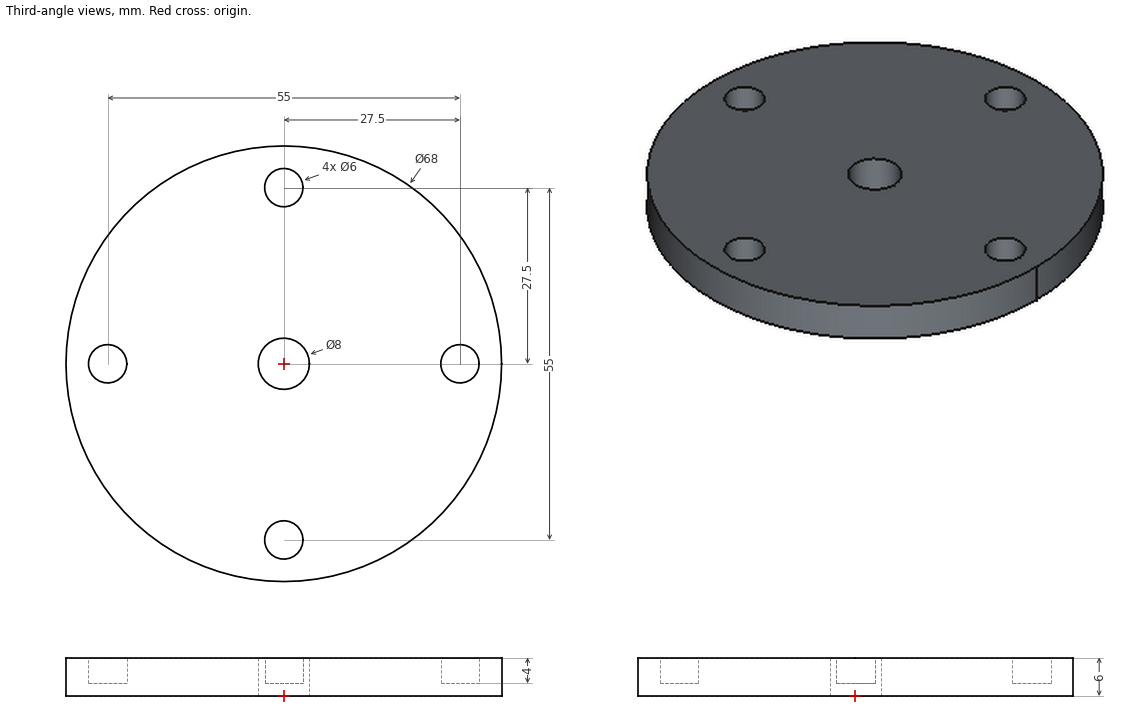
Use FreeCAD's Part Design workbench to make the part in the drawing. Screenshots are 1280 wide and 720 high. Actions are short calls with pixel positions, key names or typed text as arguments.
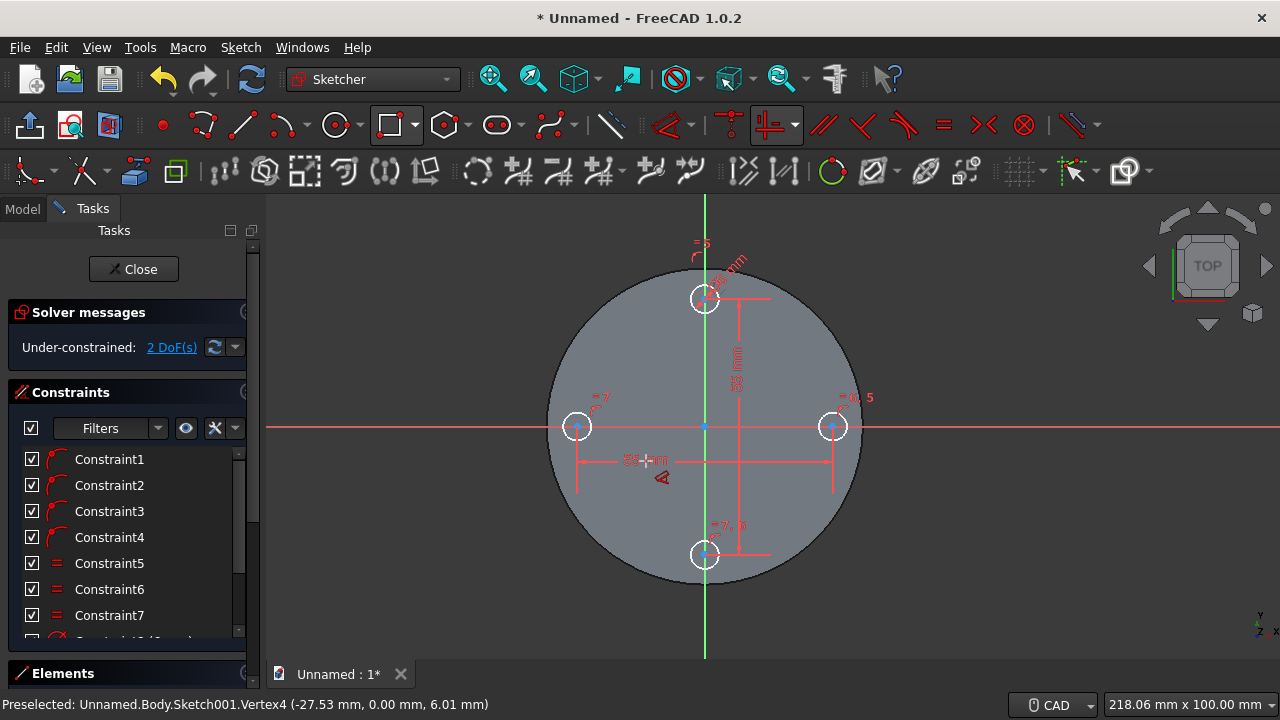
click(705, 299)
click(739, 334)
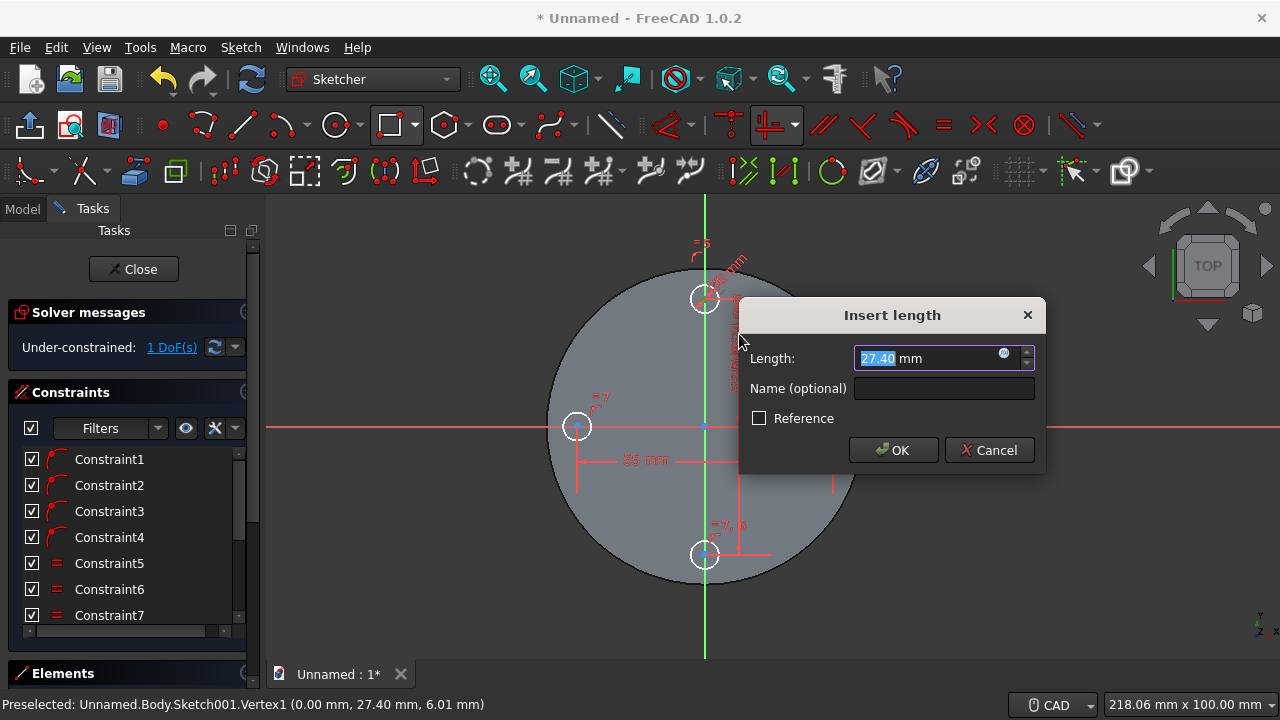
text(27.5)
key(Return)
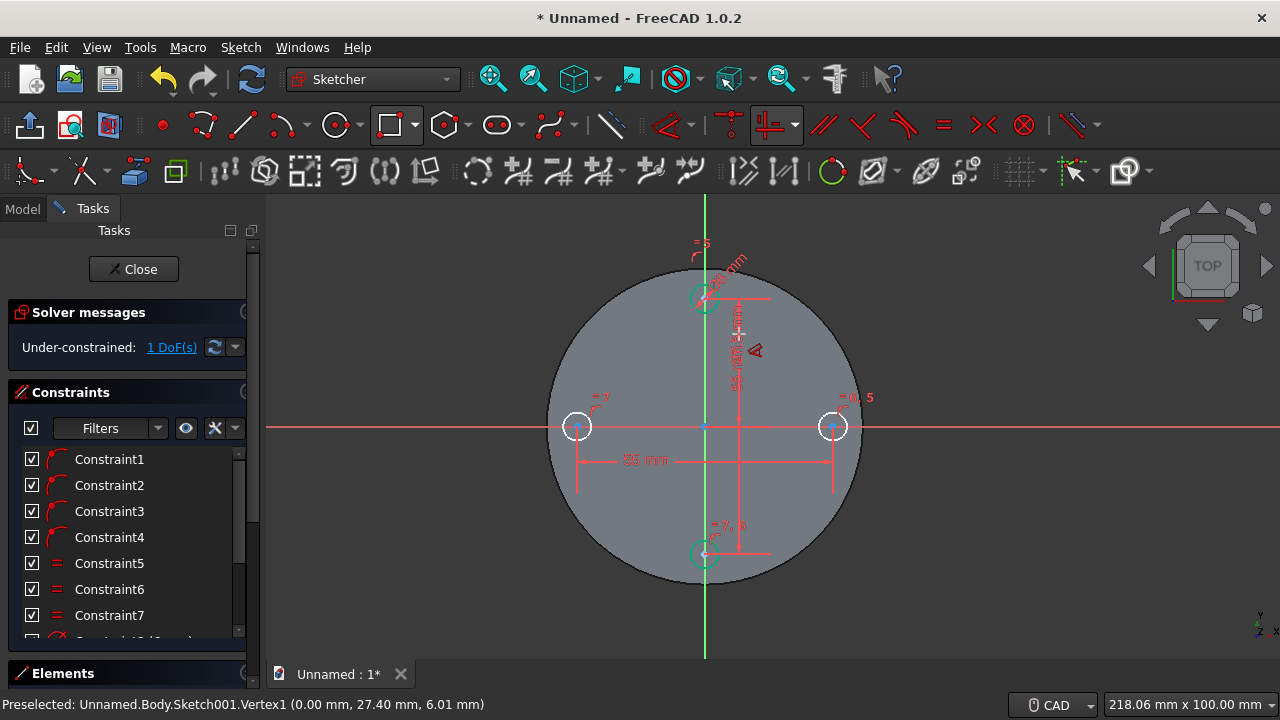
click(833, 427)
click(769, 461)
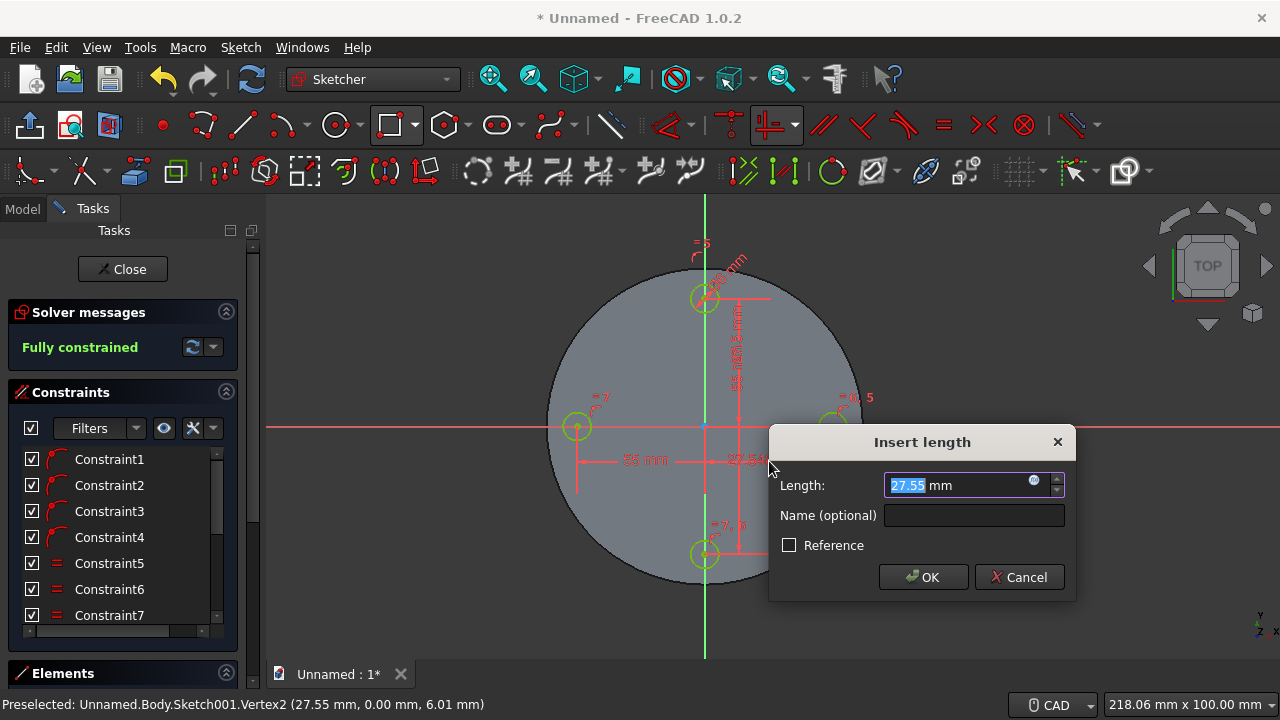
text(27.5)
key(Return)
key(Escape)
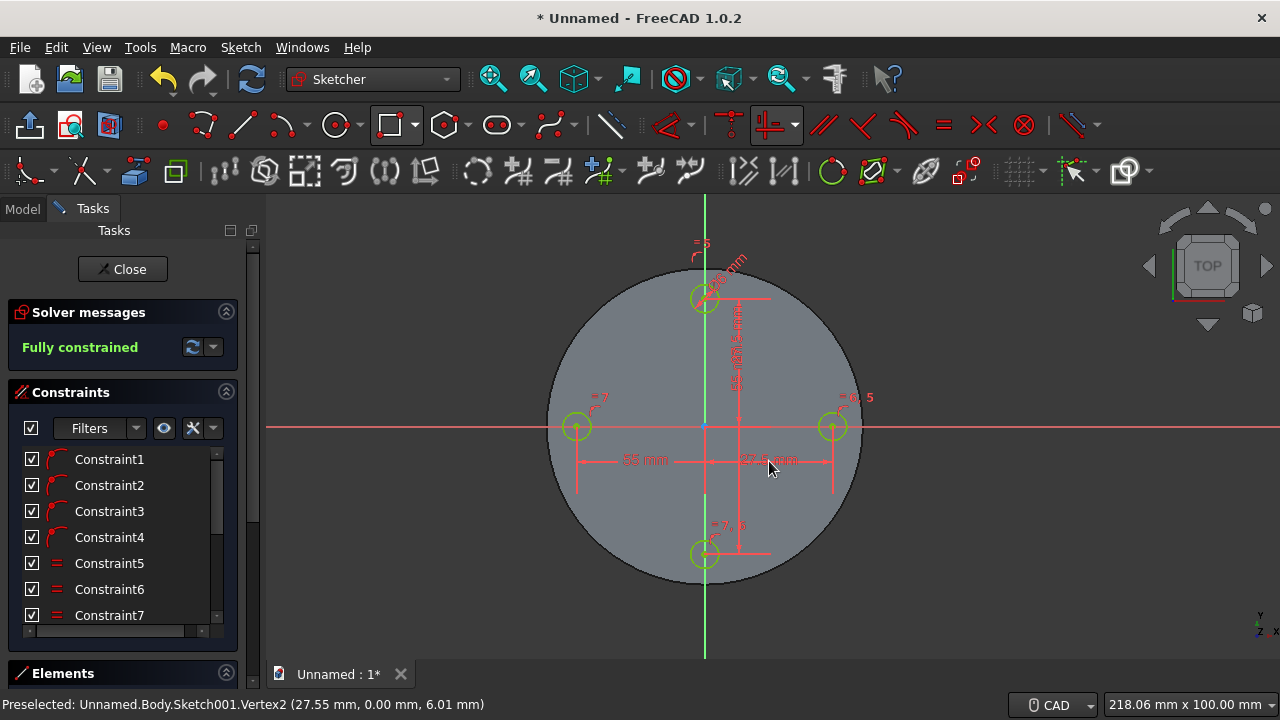
click(123, 269)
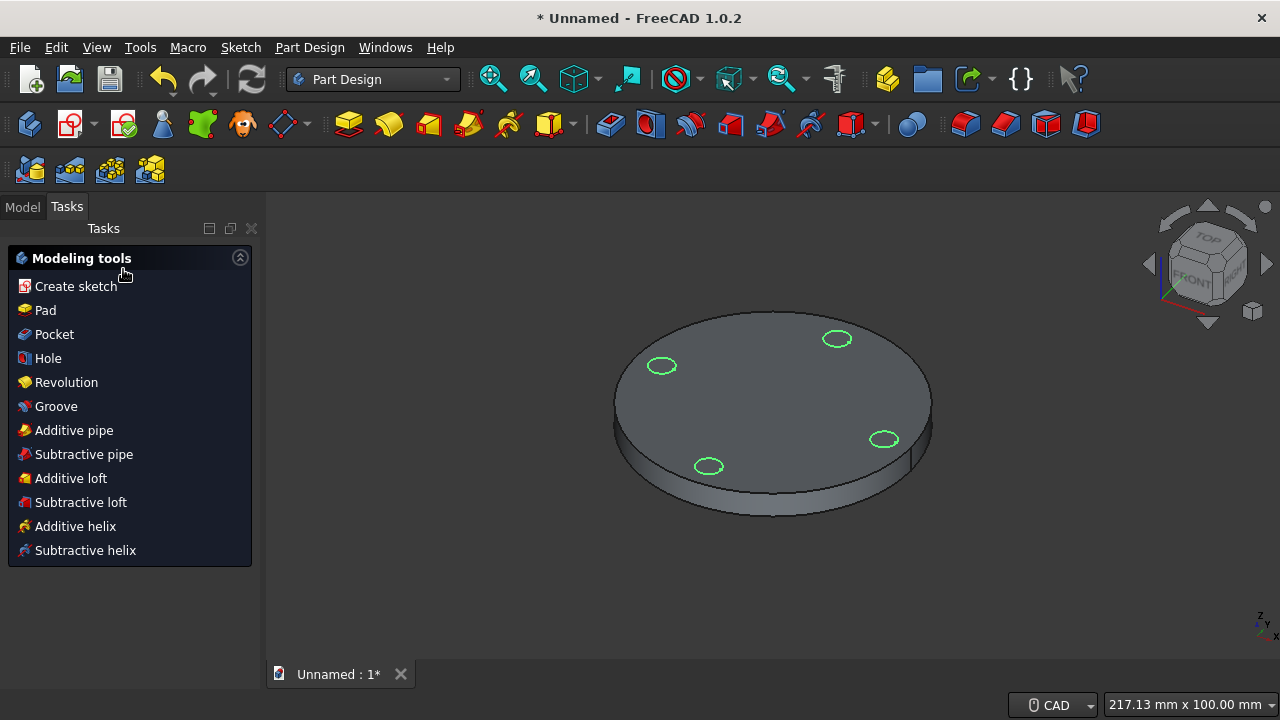
click(612, 124)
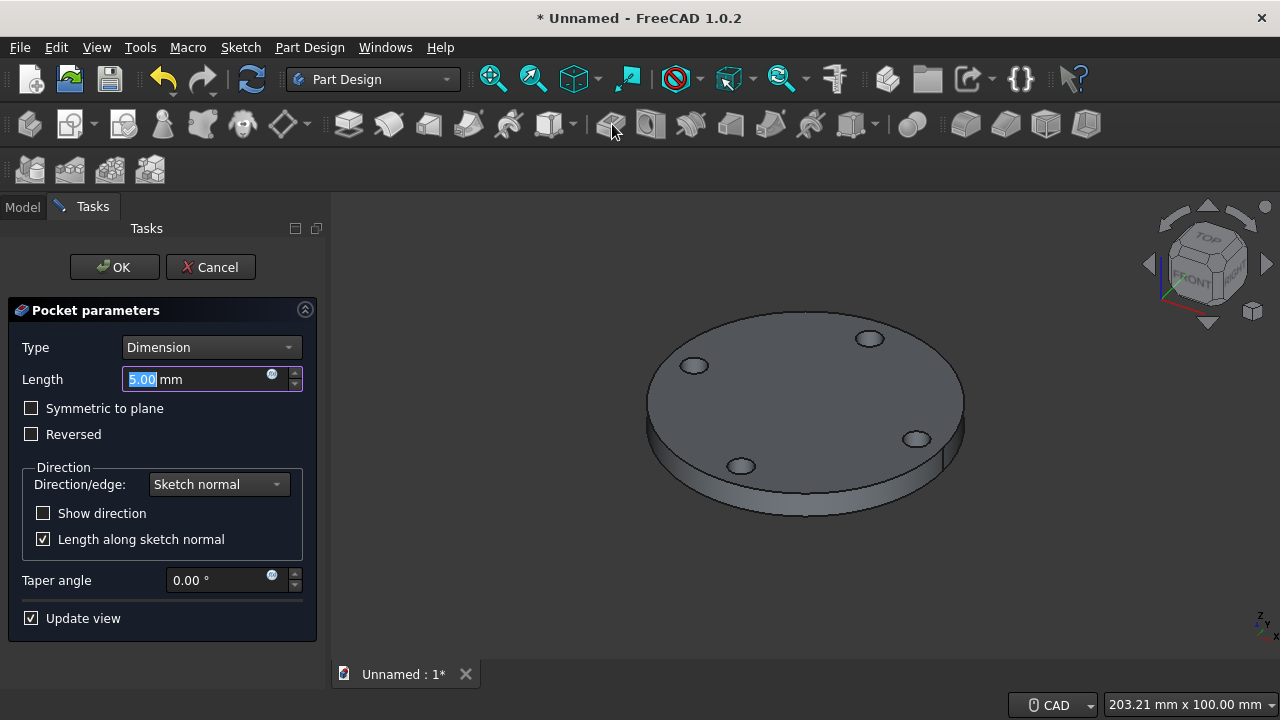
text(4)
key(Tab)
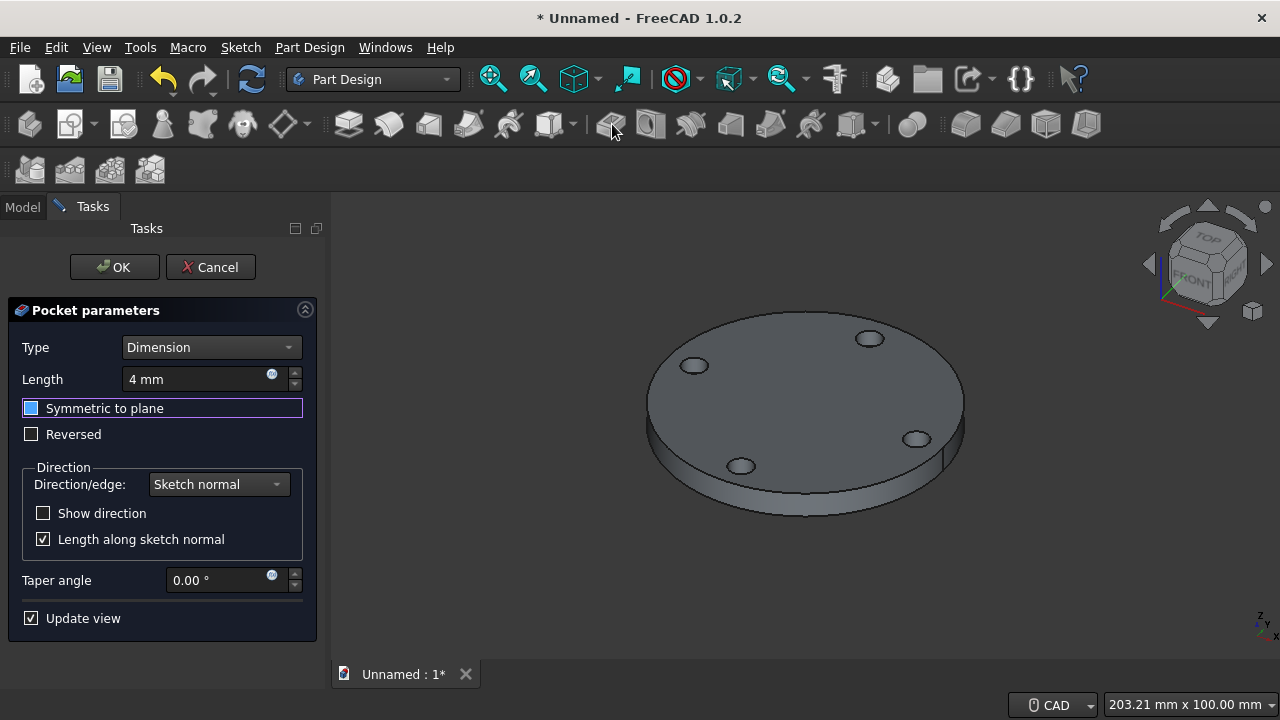
click(115, 267)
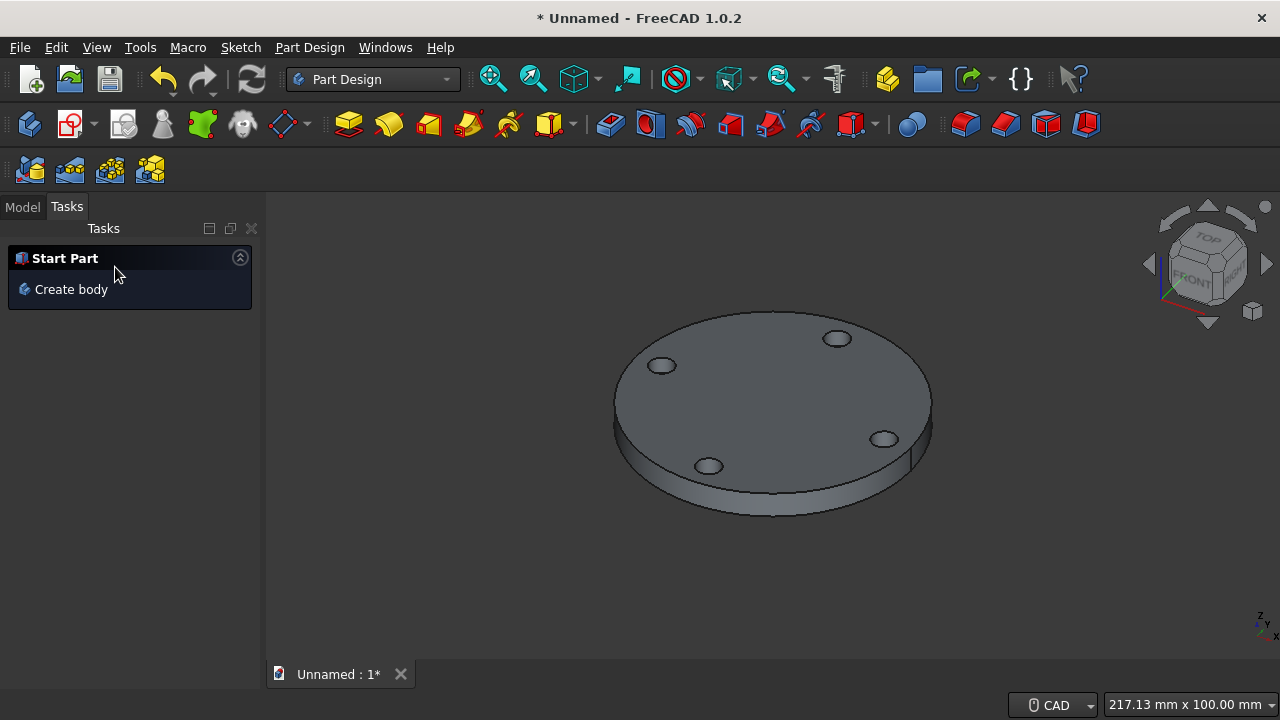
click(773, 402)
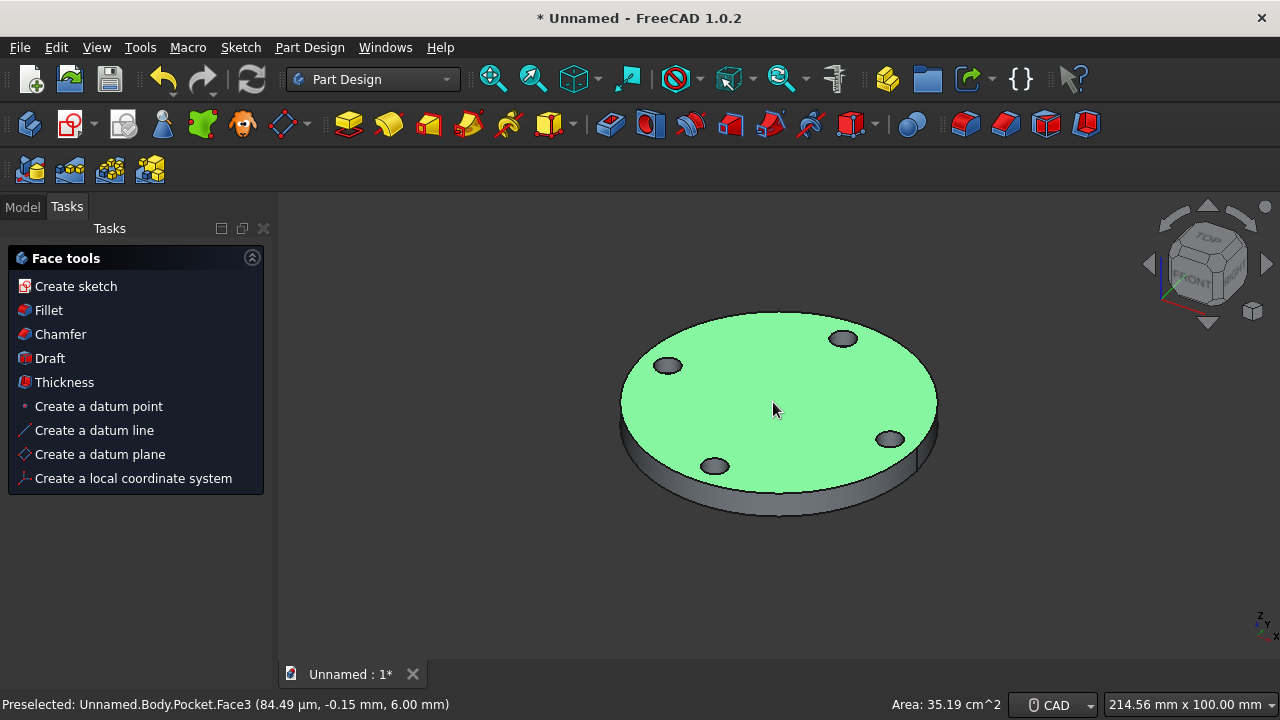
click(70, 124)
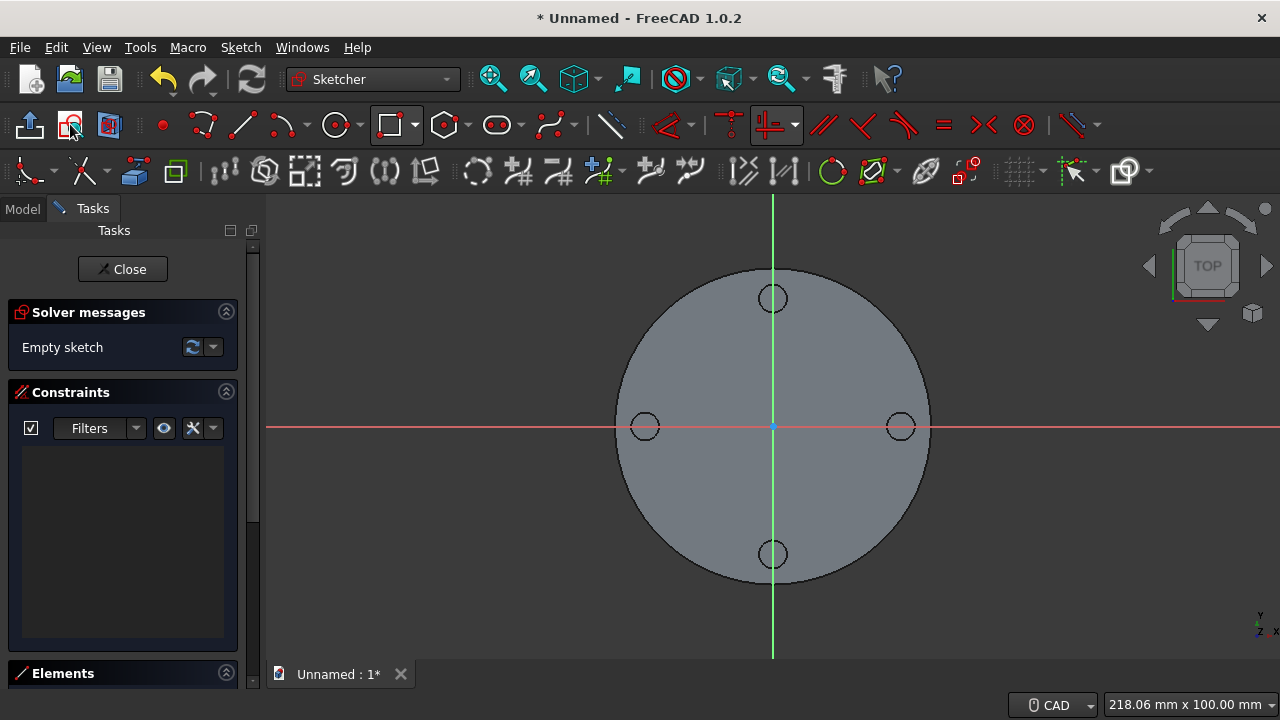
scroll(784, 426, up, 10)